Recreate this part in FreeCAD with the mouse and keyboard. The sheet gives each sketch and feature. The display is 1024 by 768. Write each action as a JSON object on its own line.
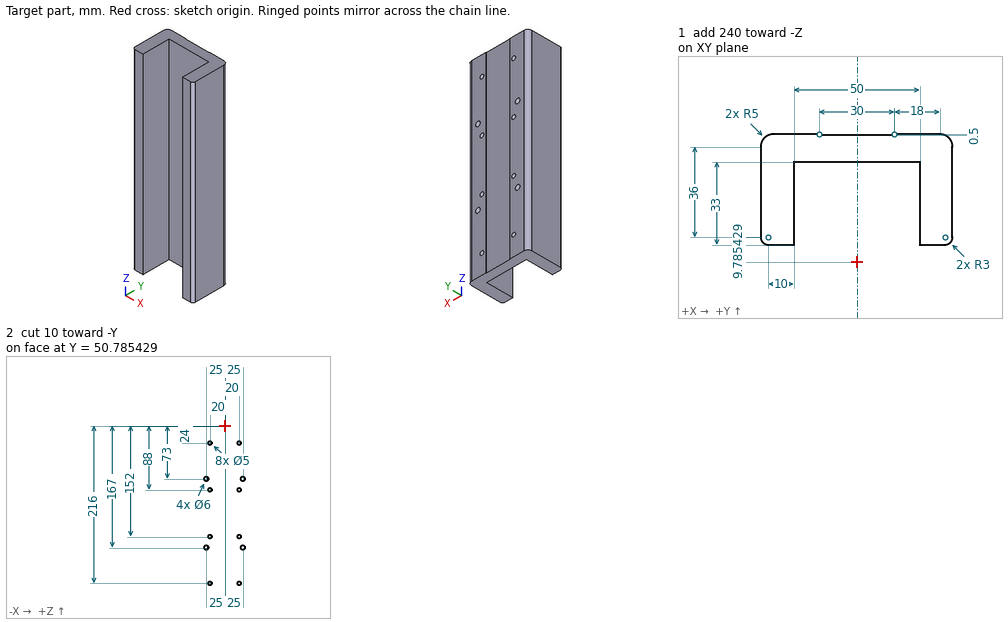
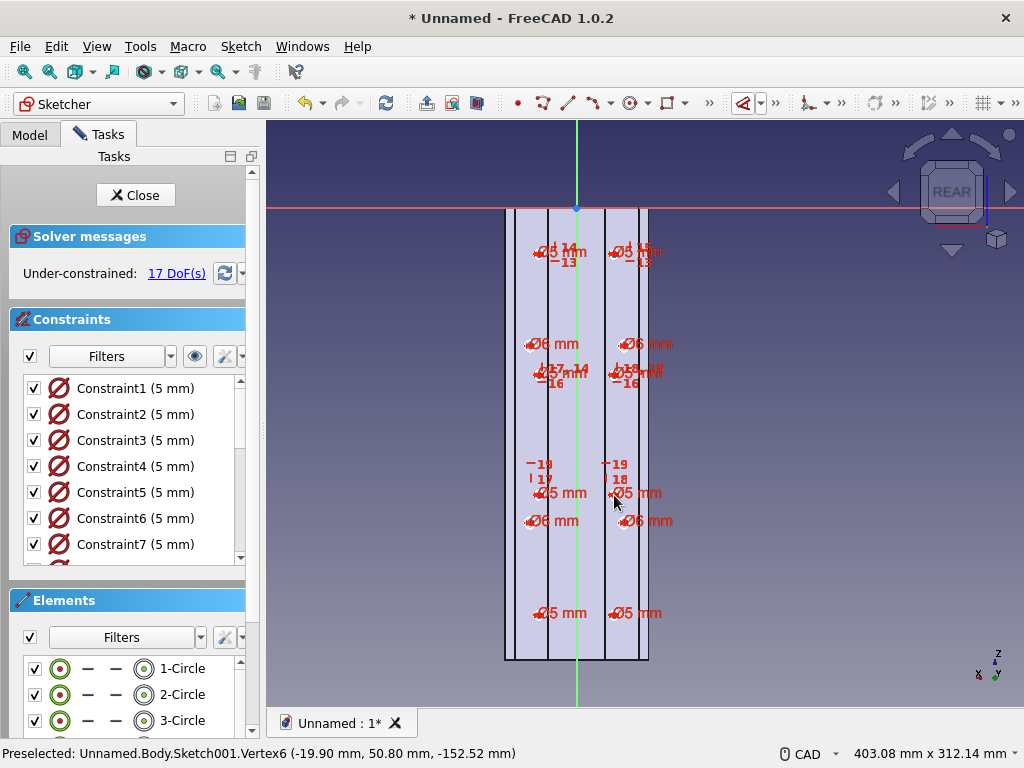
{"action": "left_click", "coordinate": [539, 495]}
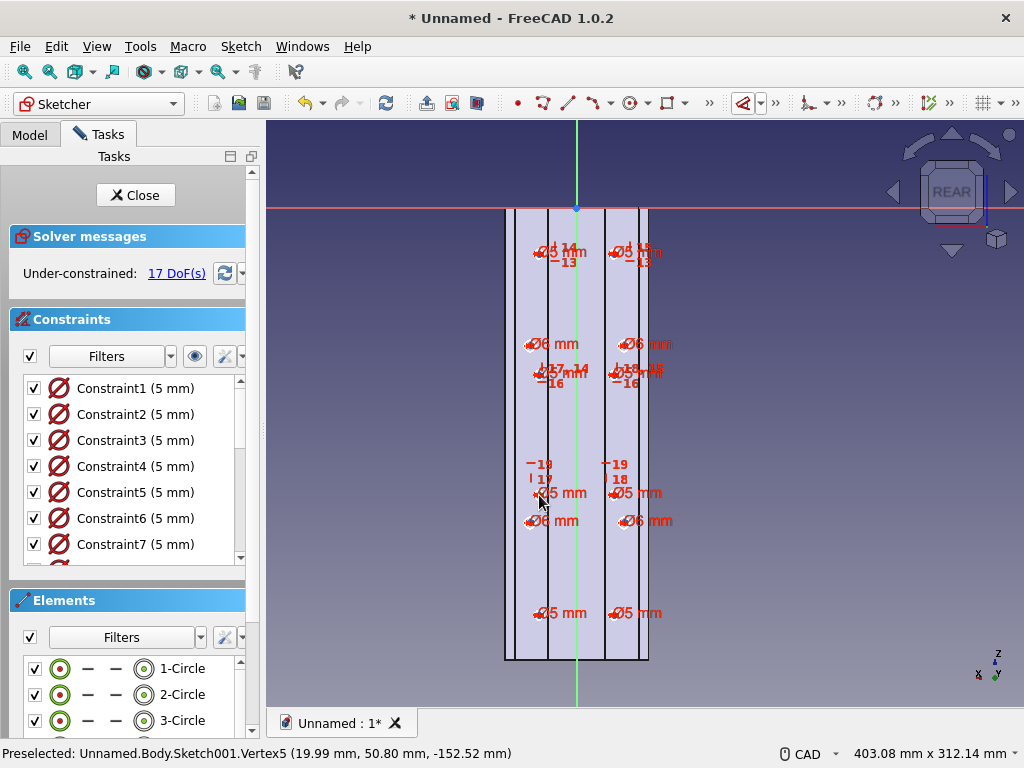
{"action": "left_click", "coordinate": [539, 615]}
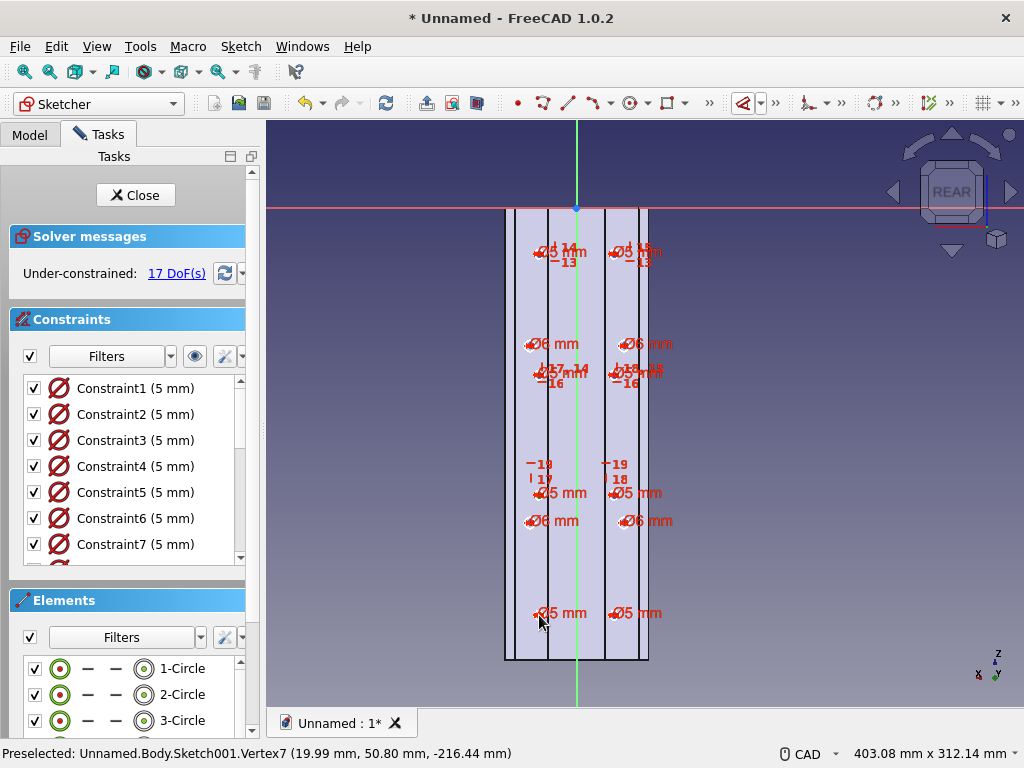
{"action": "key", "text": "v"}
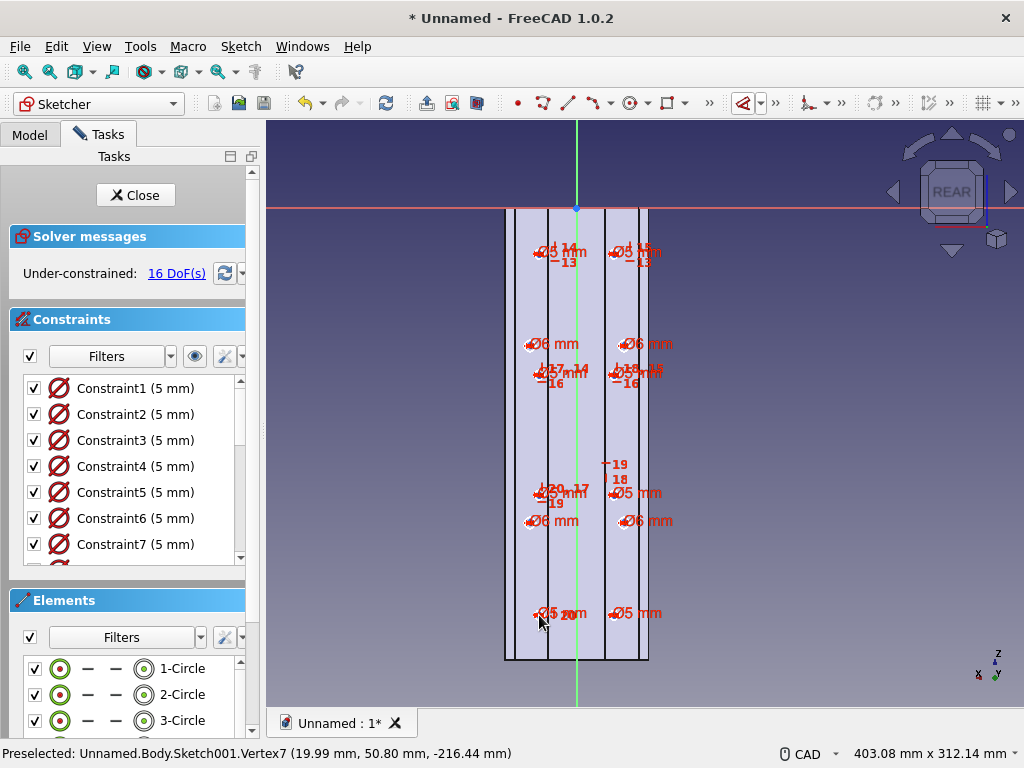
{"action": "left_click", "coordinate": [614, 495]}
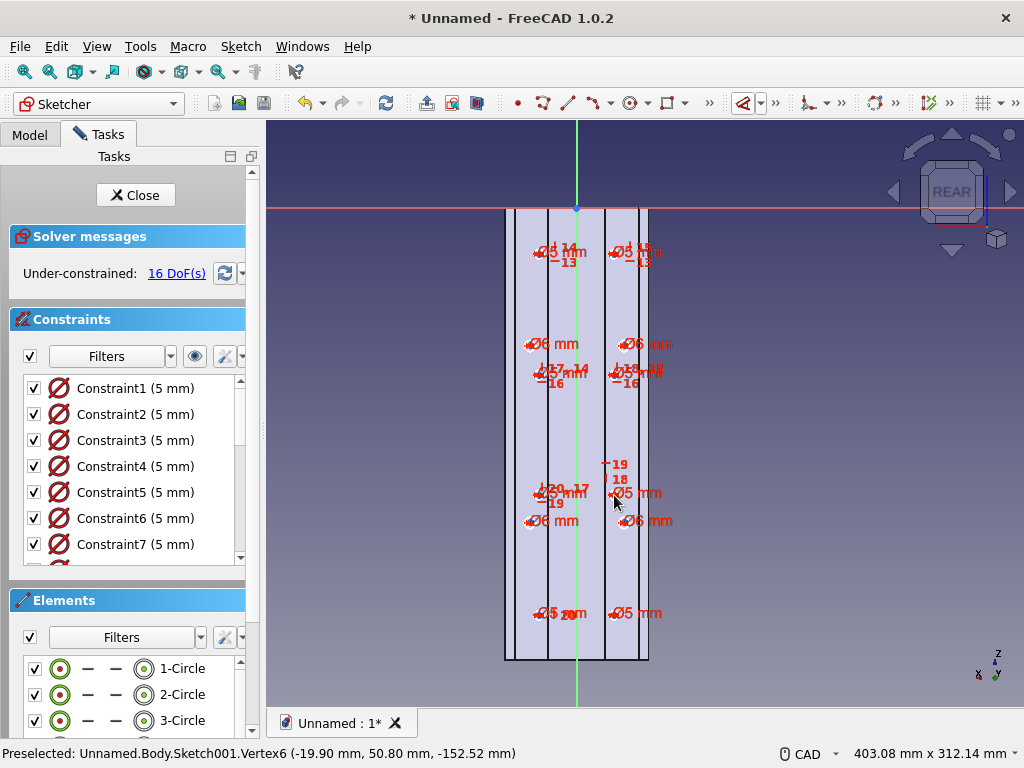
{"action": "left_click", "coordinate": [614, 615]}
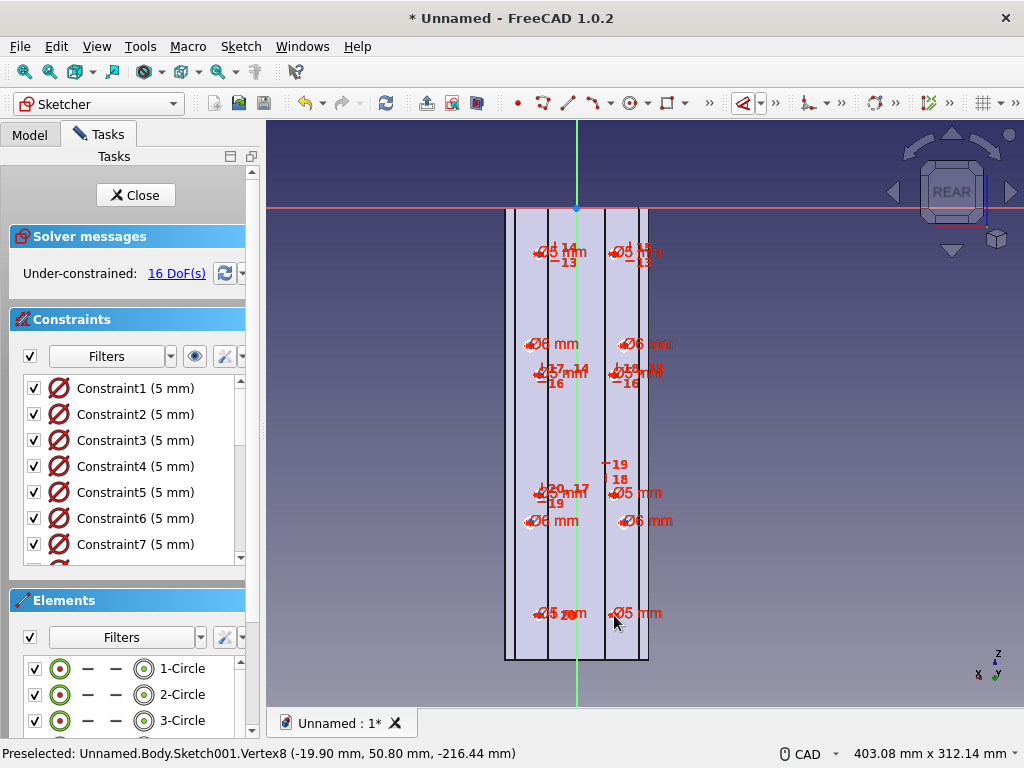
{"action": "key", "text": "v"}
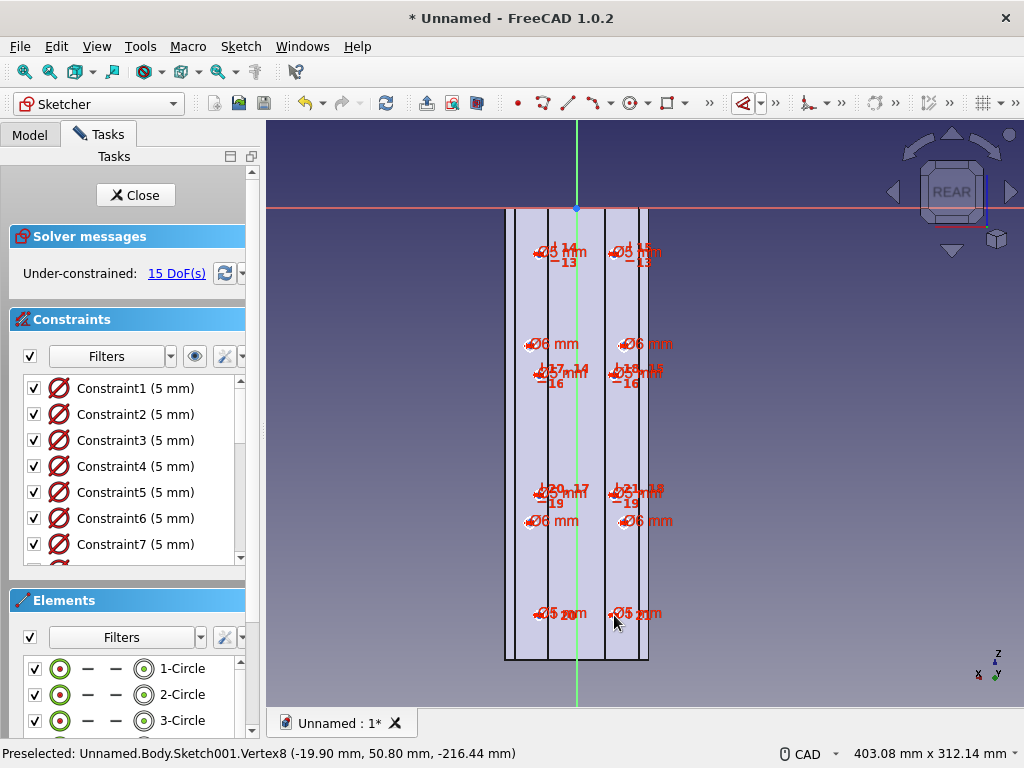
{"action": "left_click", "coordinate": [539, 615]}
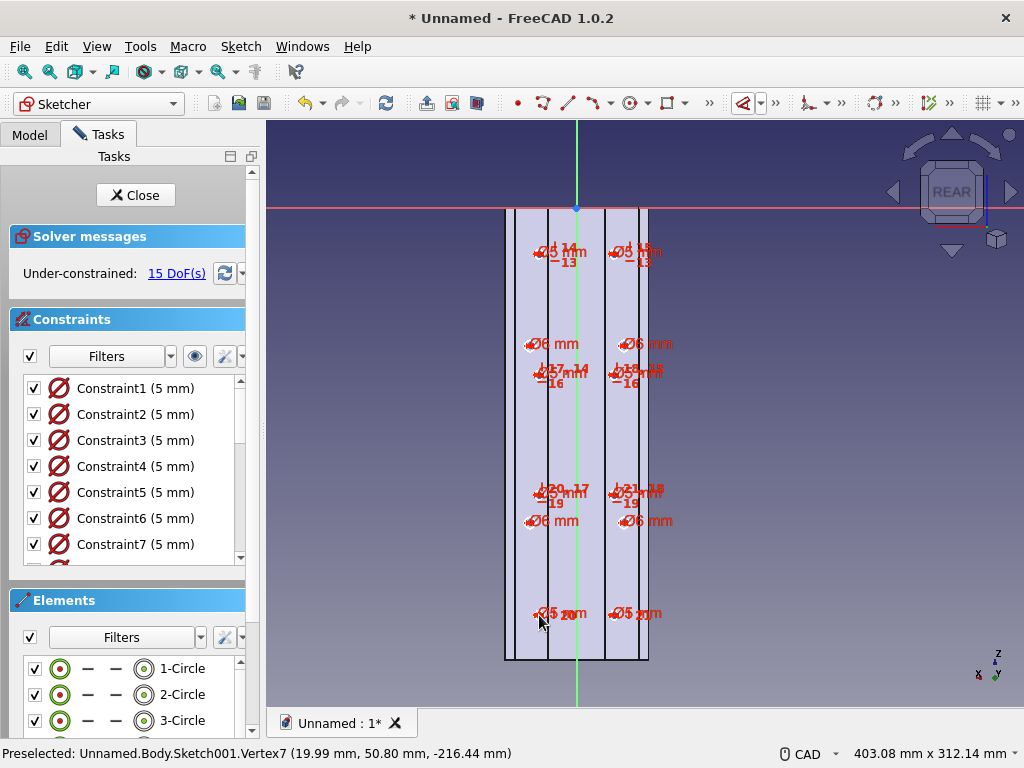
{"action": "left_click", "coordinate": [614, 615]}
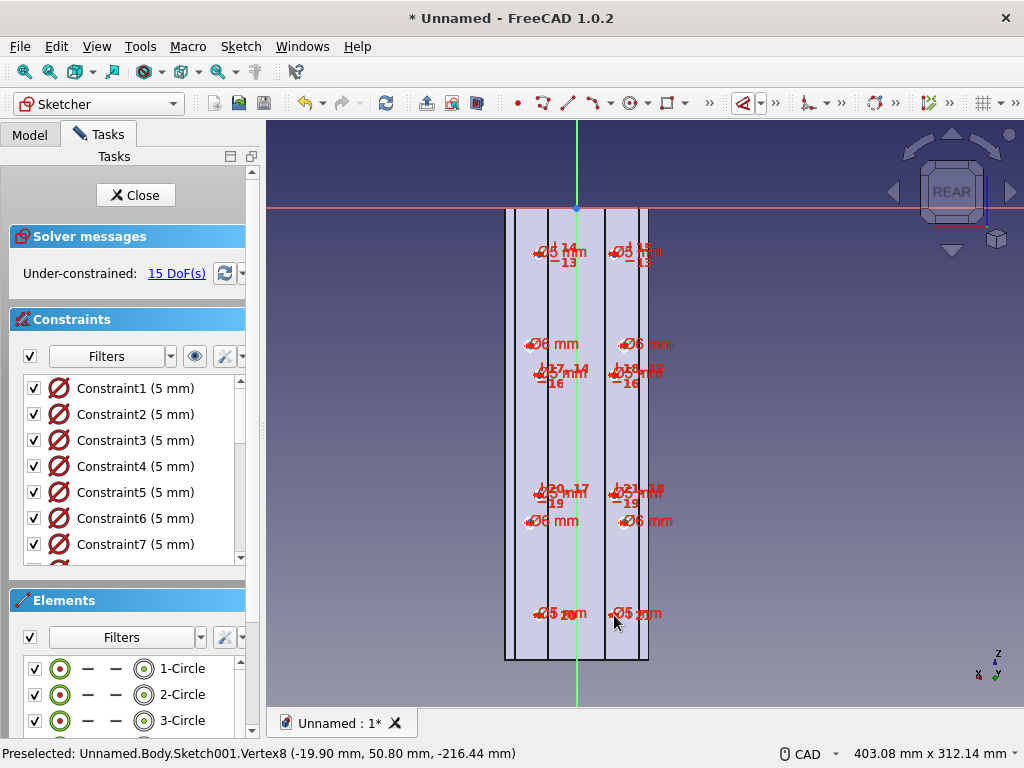
{"action": "key", "text": "h"}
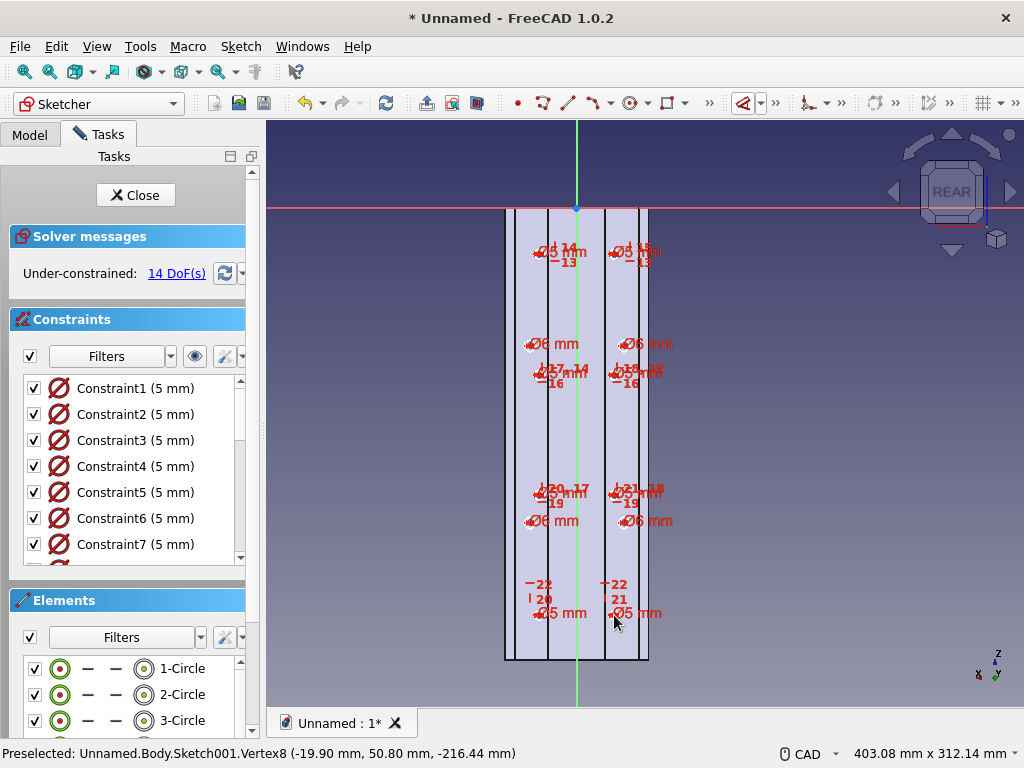
{"action": "left_click", "coordinate": [530, 346]}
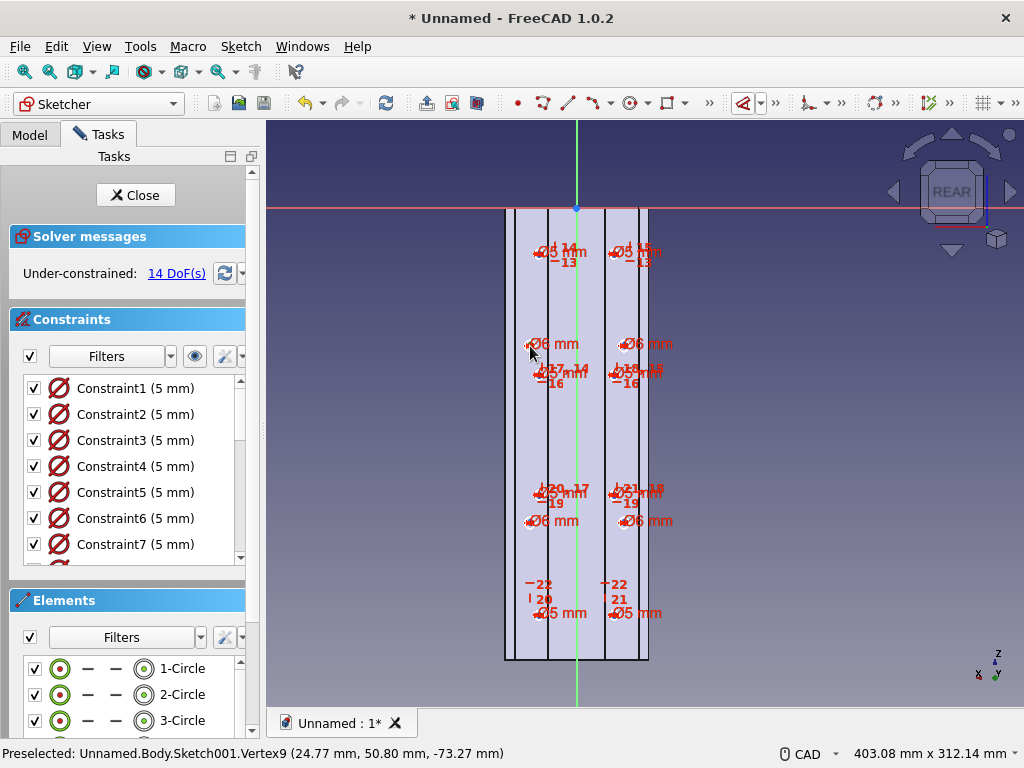
{"action": "left_click", "coordinate": [624, 346]}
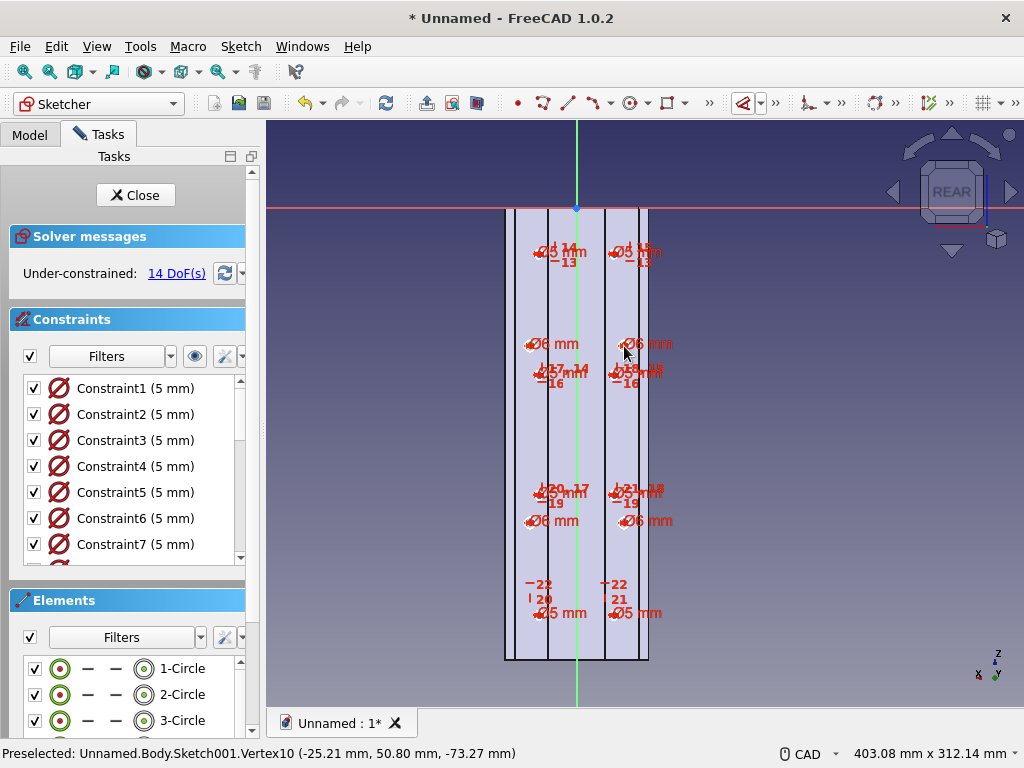
{"action": "key", "text": "h"}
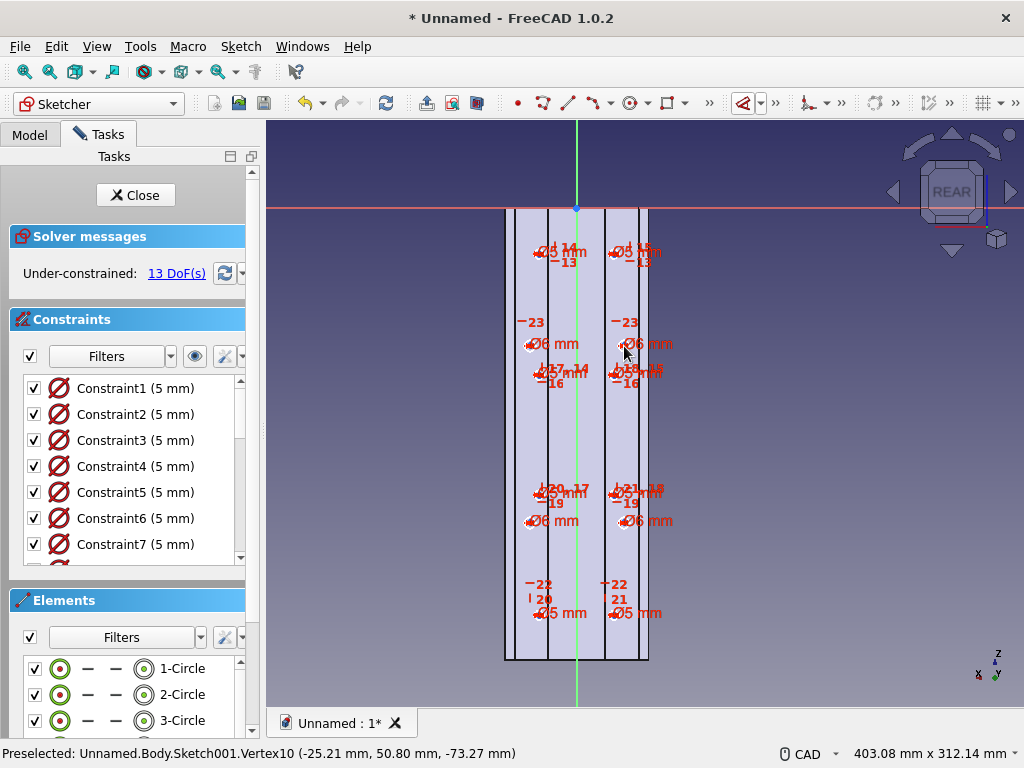
{"action": "left_click", "coordinate": [530, 523]}